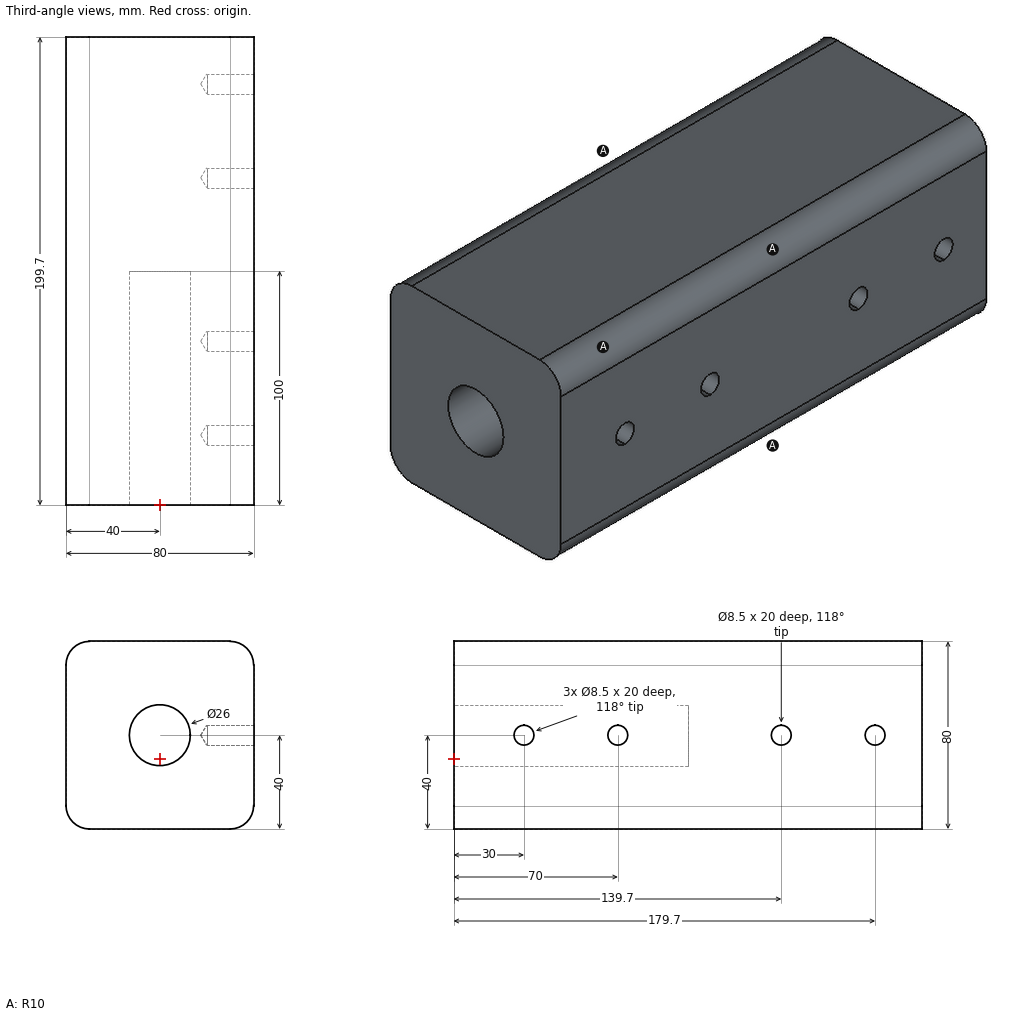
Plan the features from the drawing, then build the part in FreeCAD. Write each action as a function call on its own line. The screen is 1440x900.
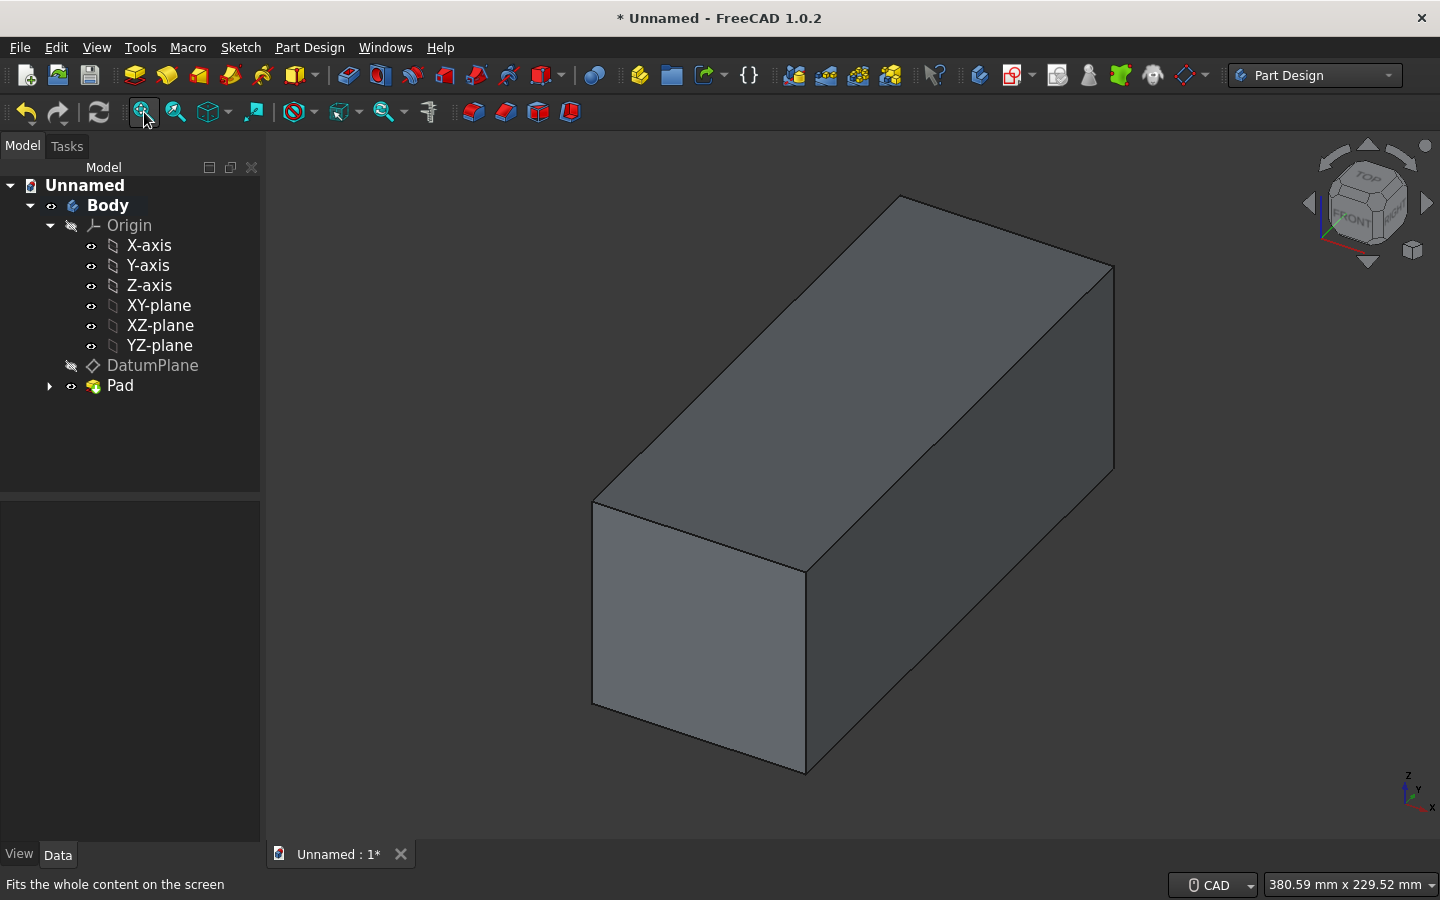
click(1048, 432)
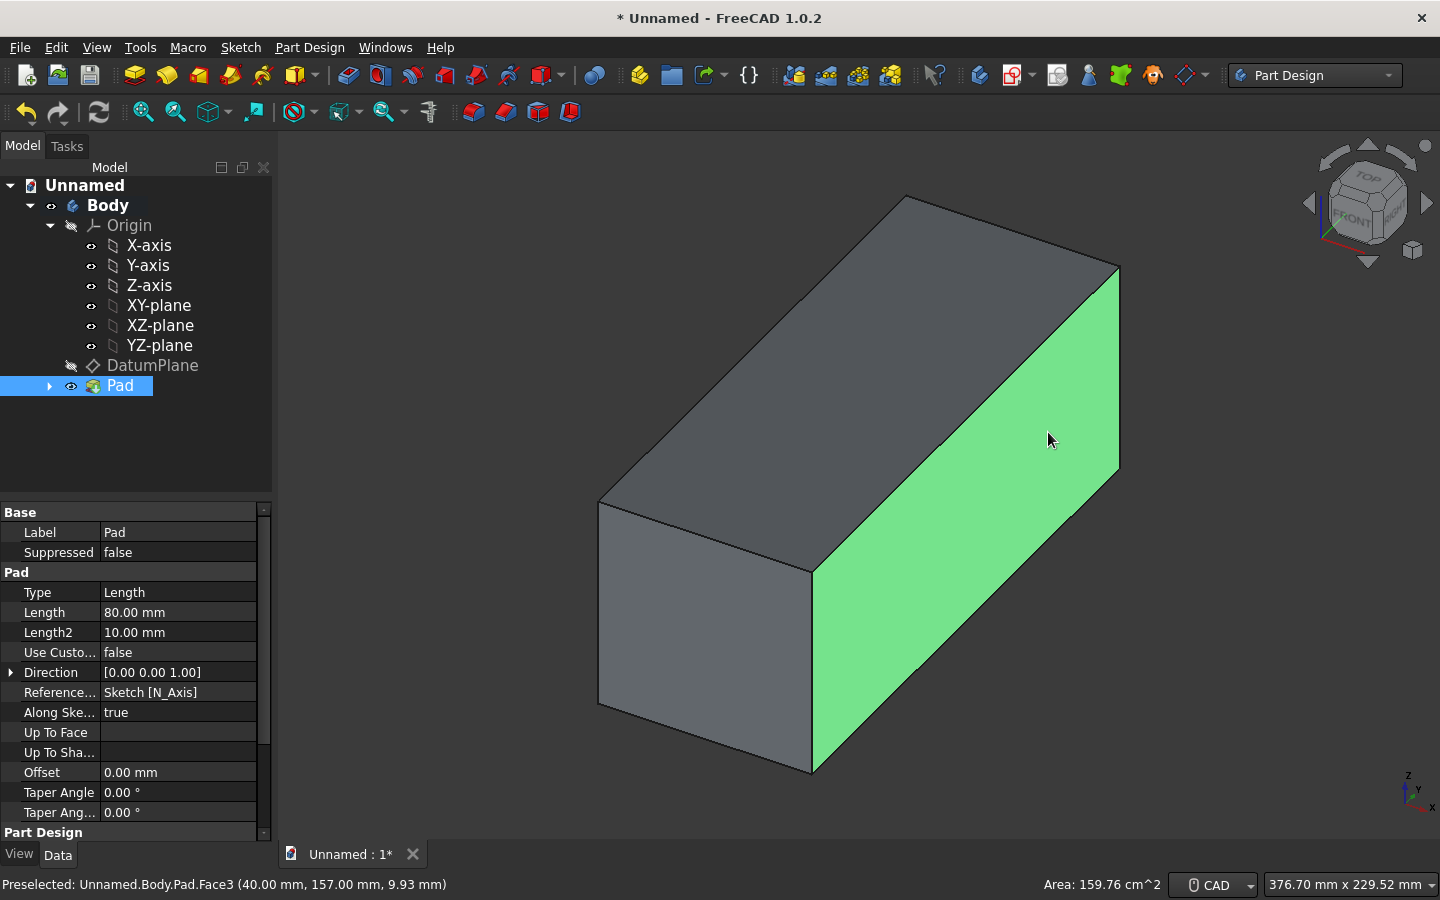
click(1012, 76)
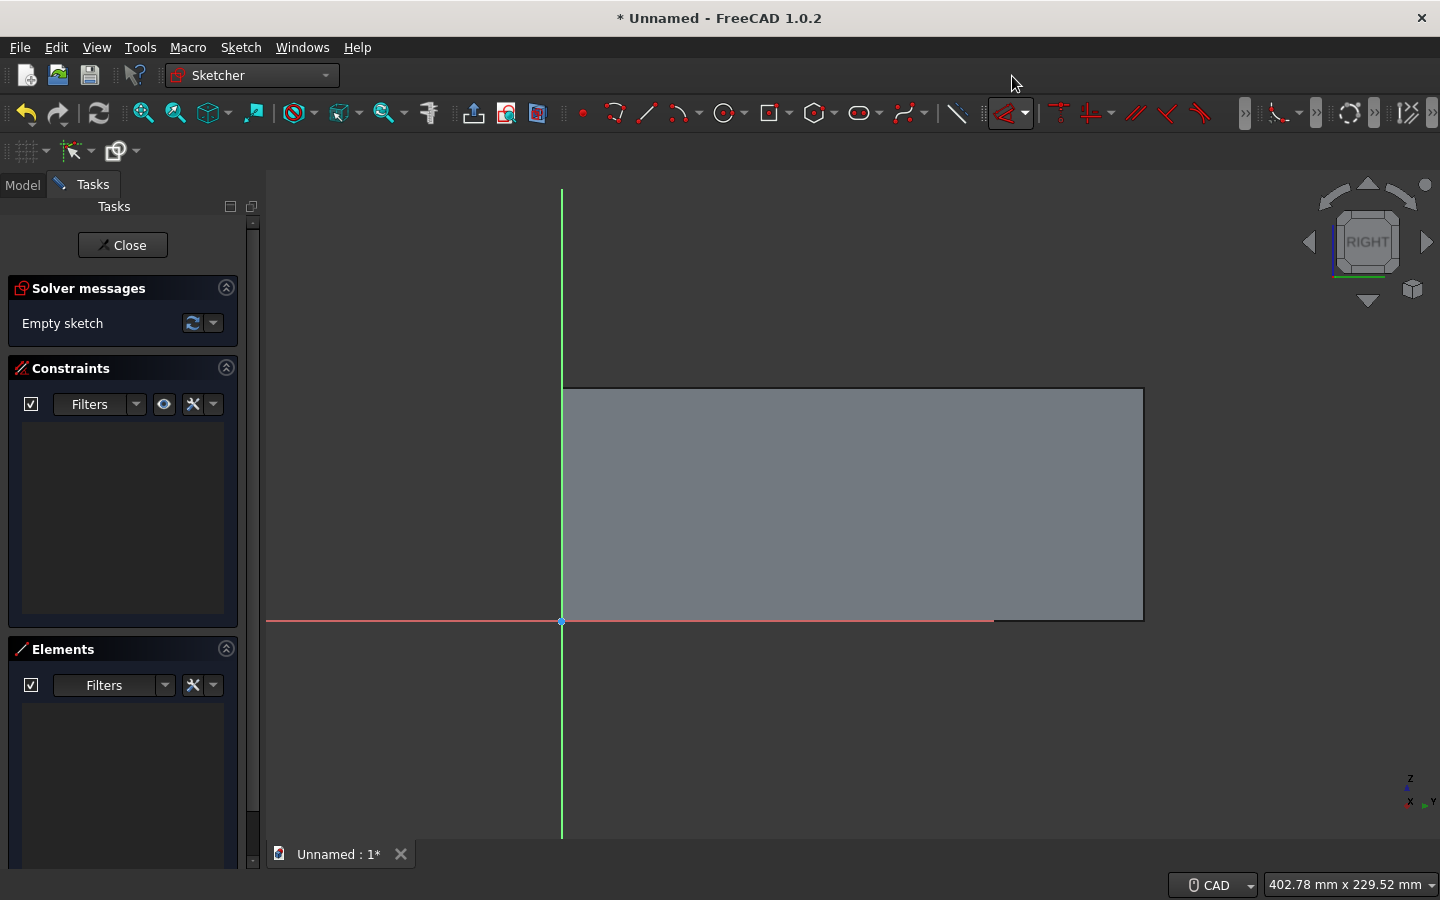
click(724, 114)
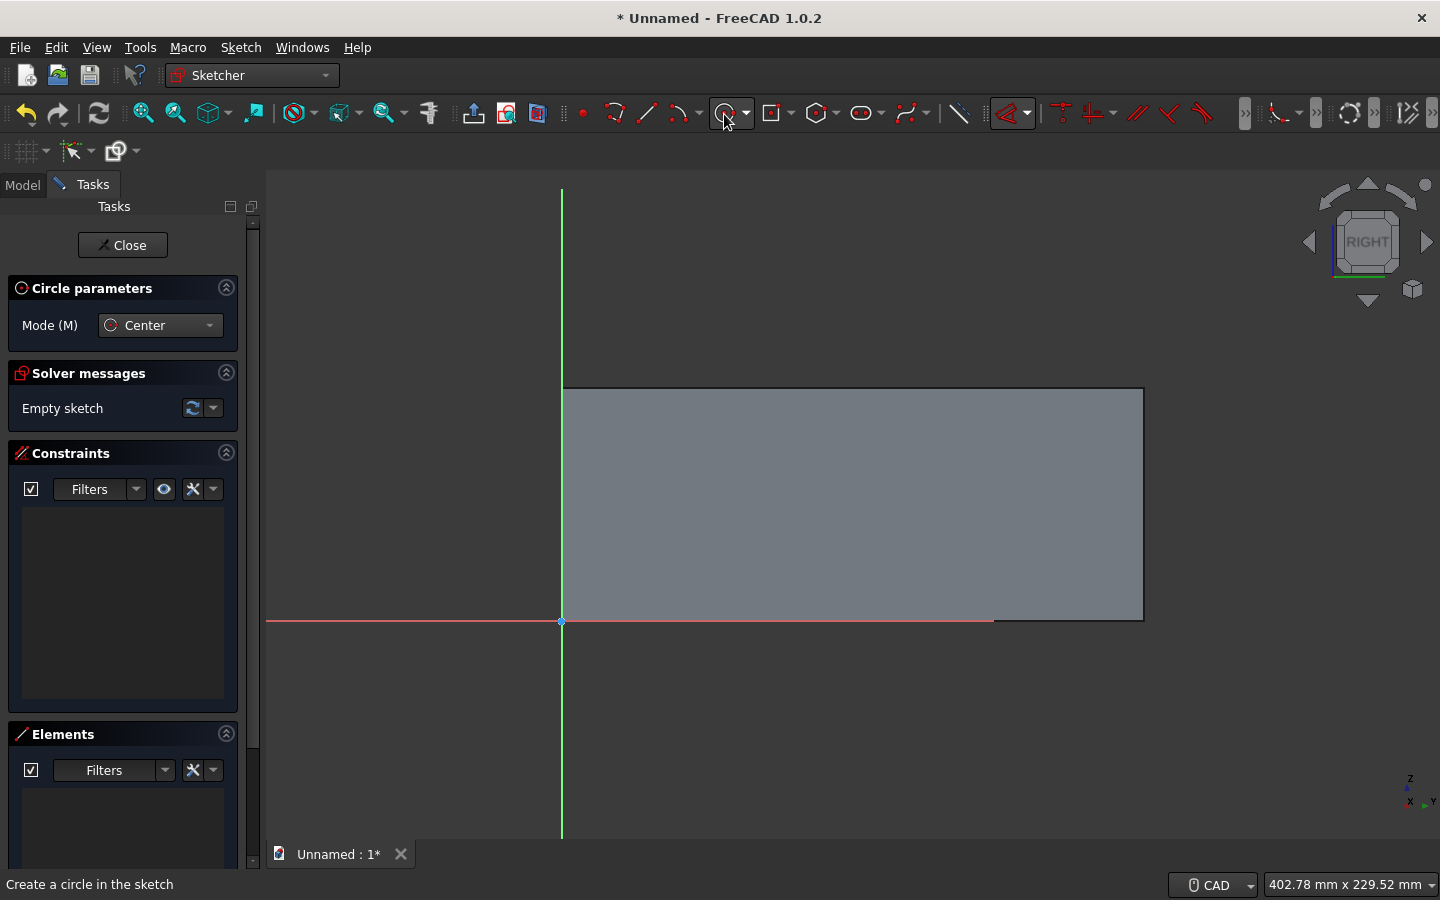
scroll(649, 505, up, 4)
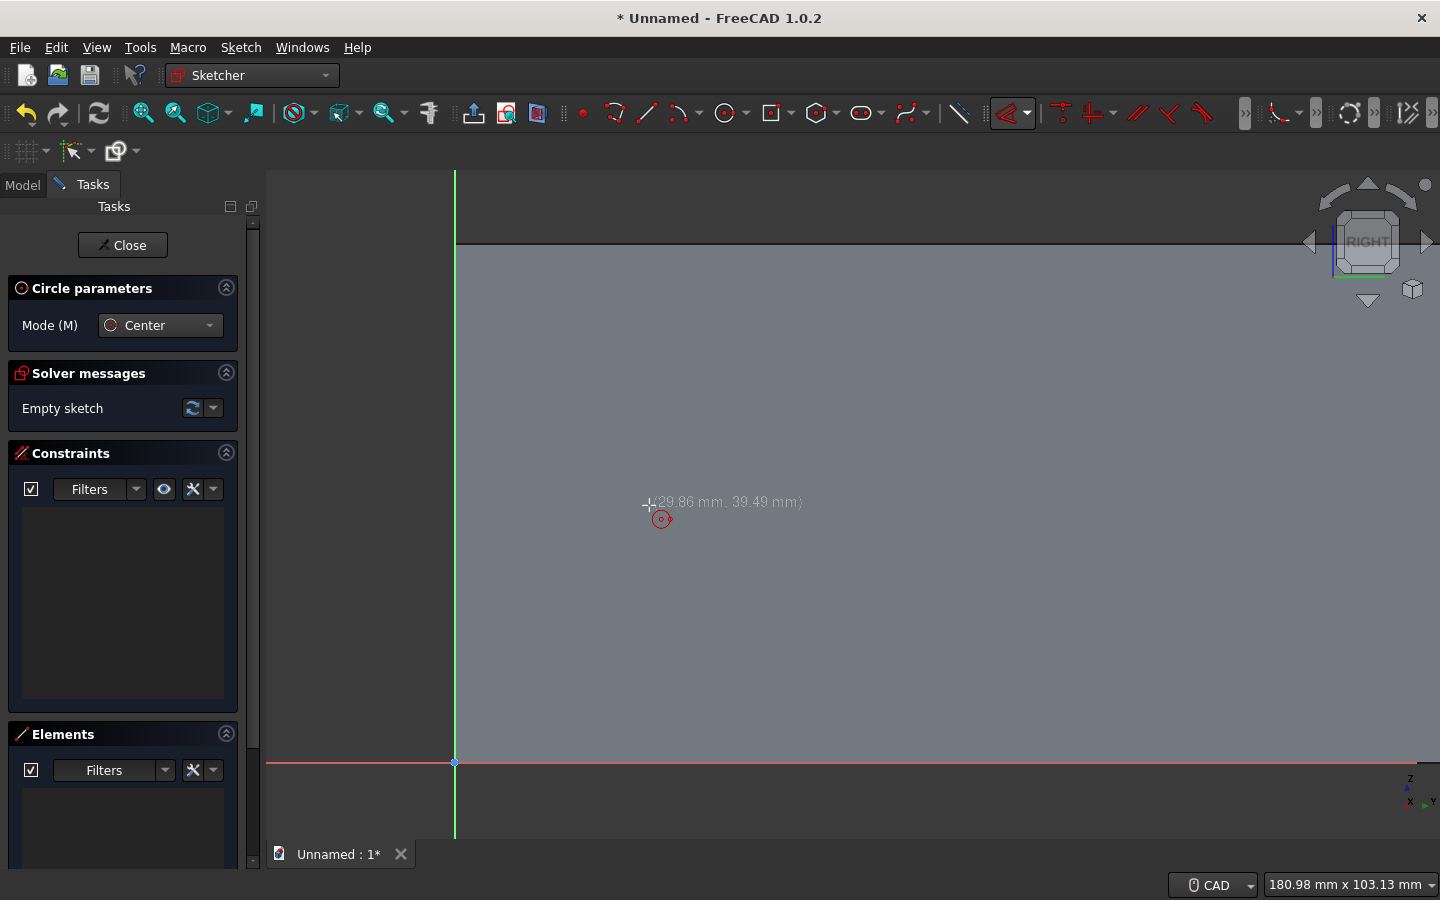
click(649, 503)
click(669, 484)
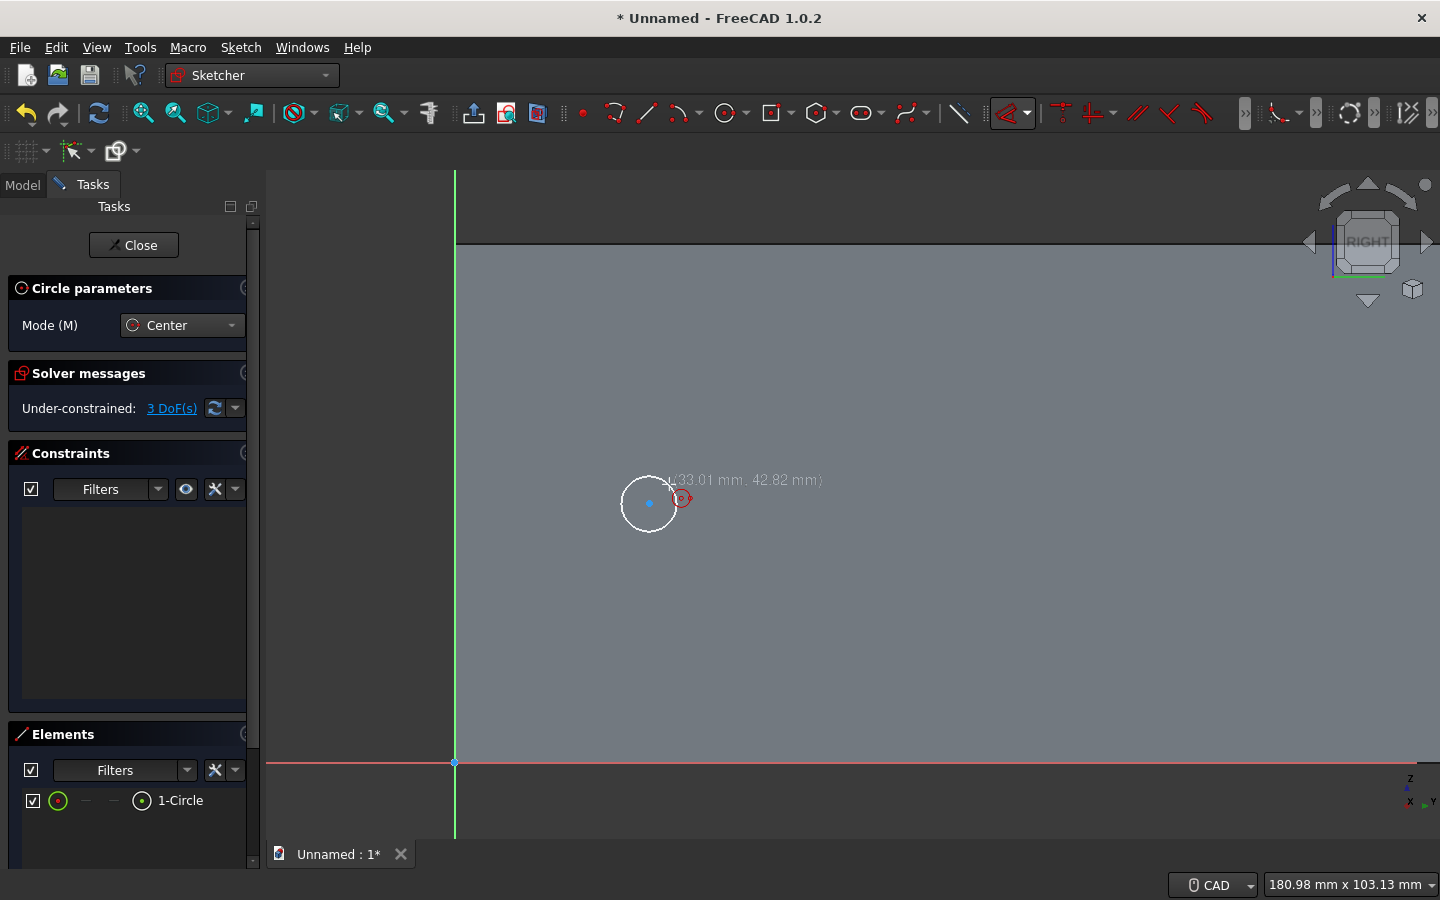
scroll(460, 365, down, 3)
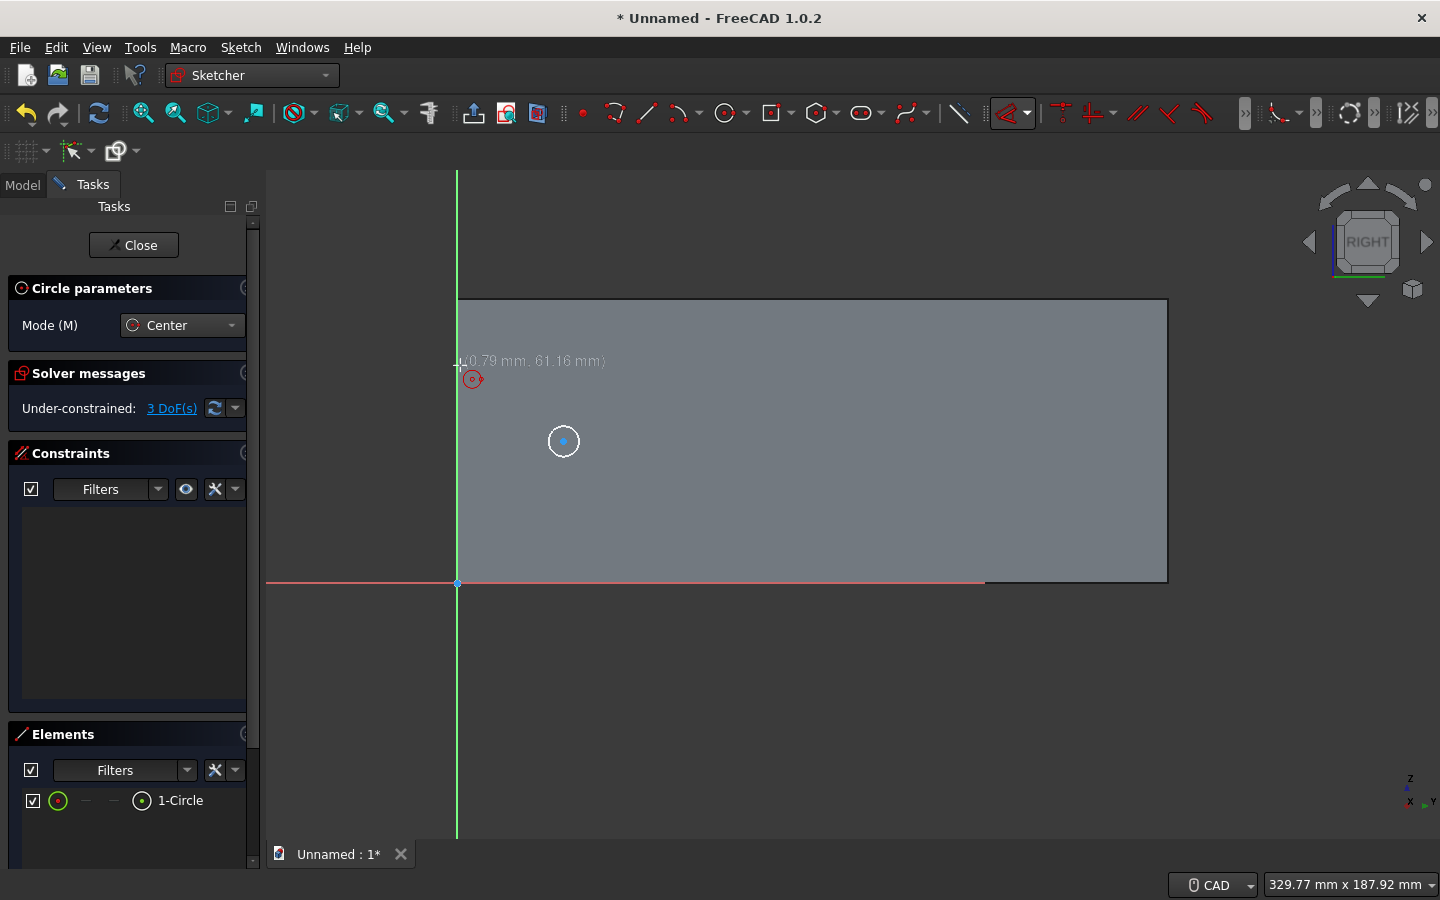
scroll(1097, 441, up, 3)